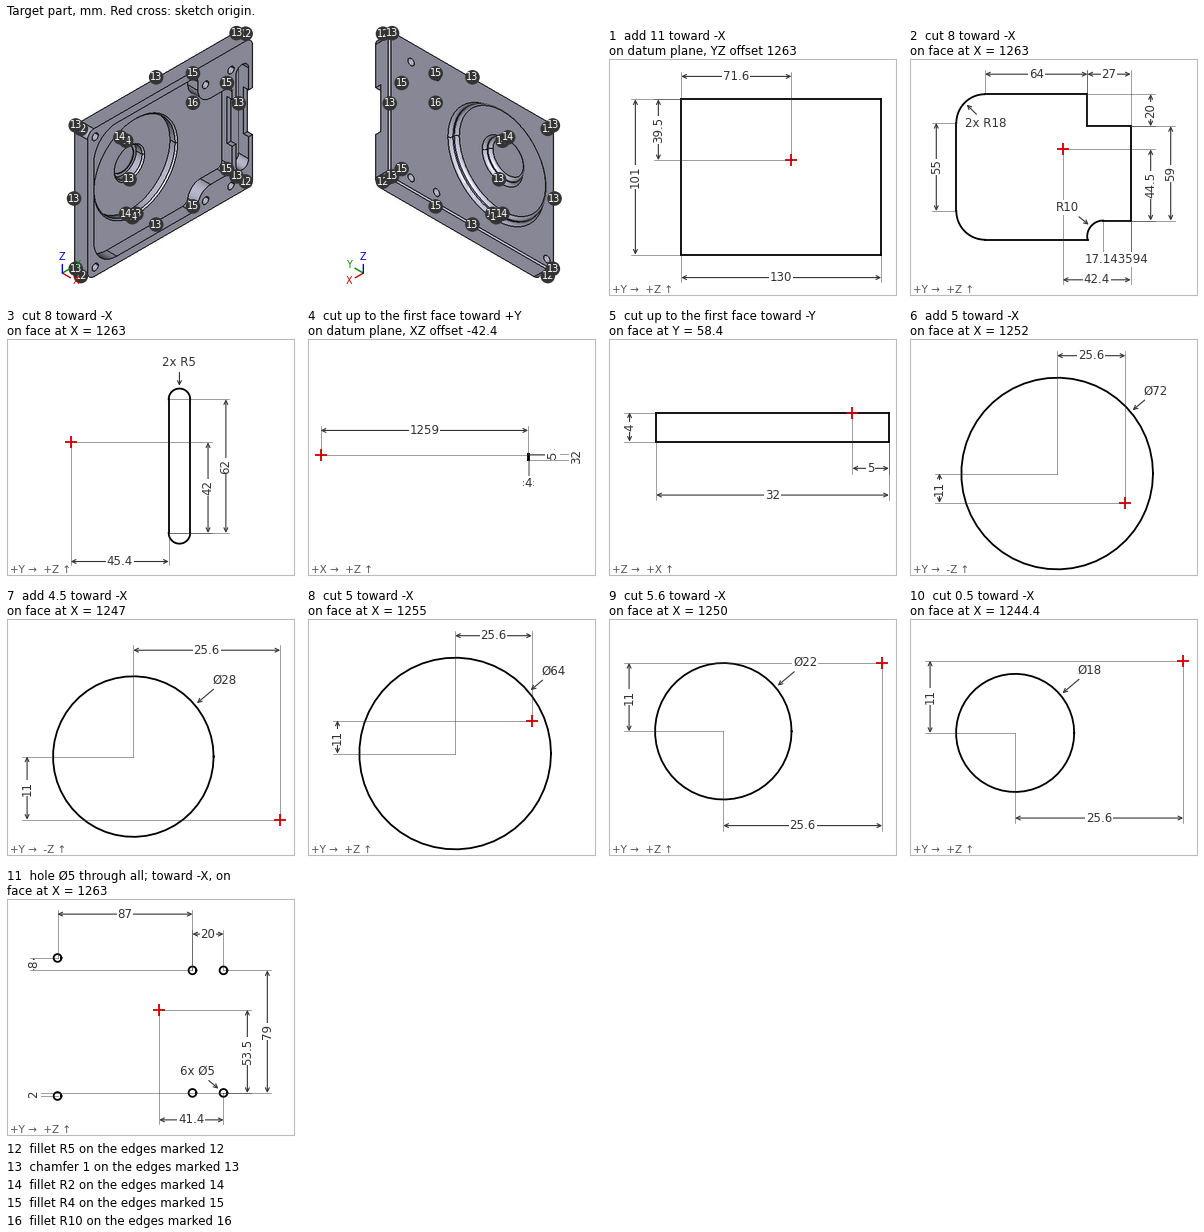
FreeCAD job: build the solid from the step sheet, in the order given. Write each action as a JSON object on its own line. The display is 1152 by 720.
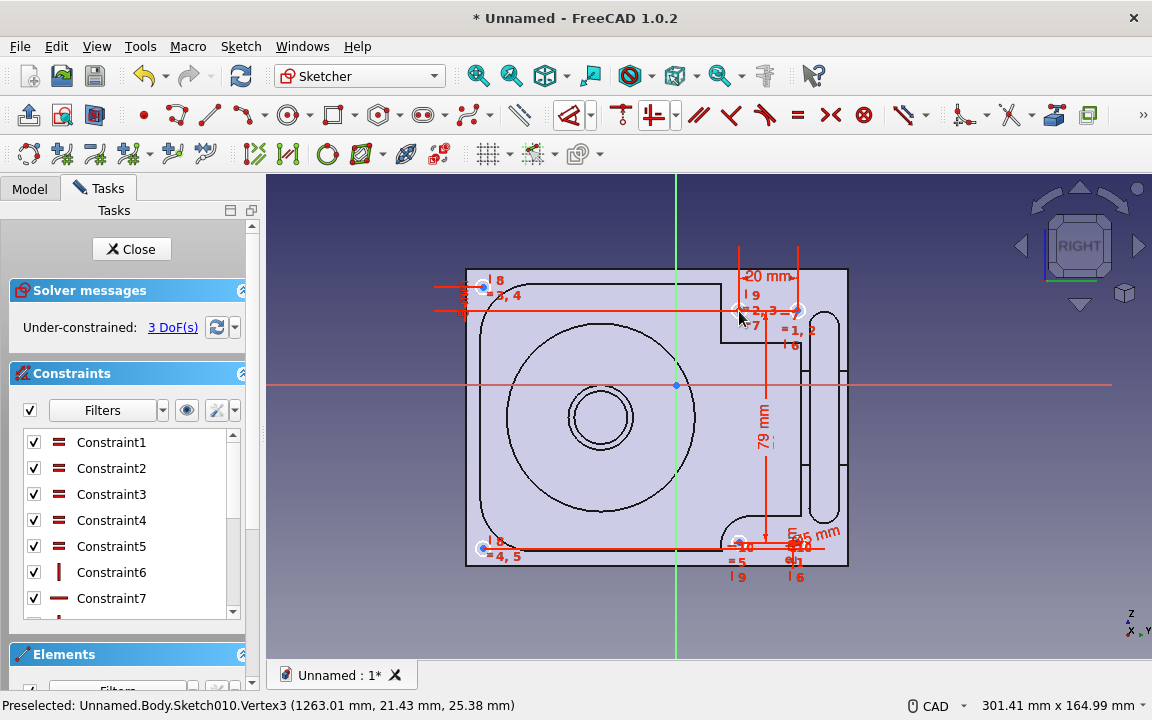
{"action": "left_click", "coordinate": [483, 287]}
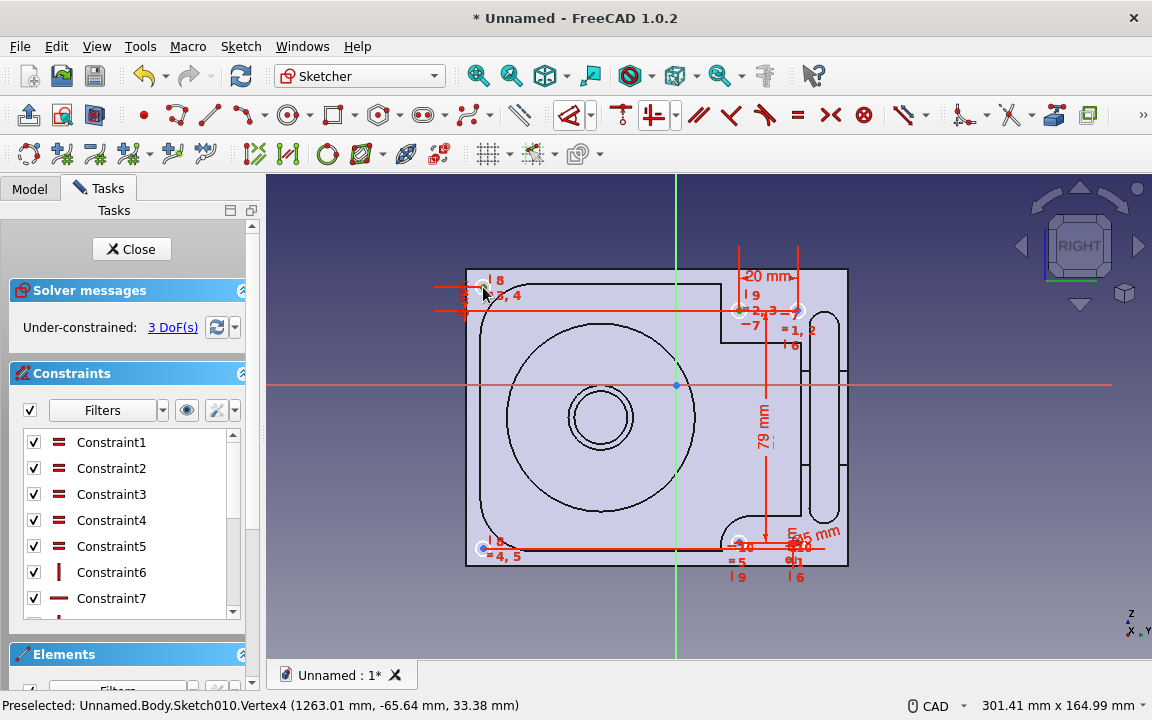
{"action": "key", "text": "l"}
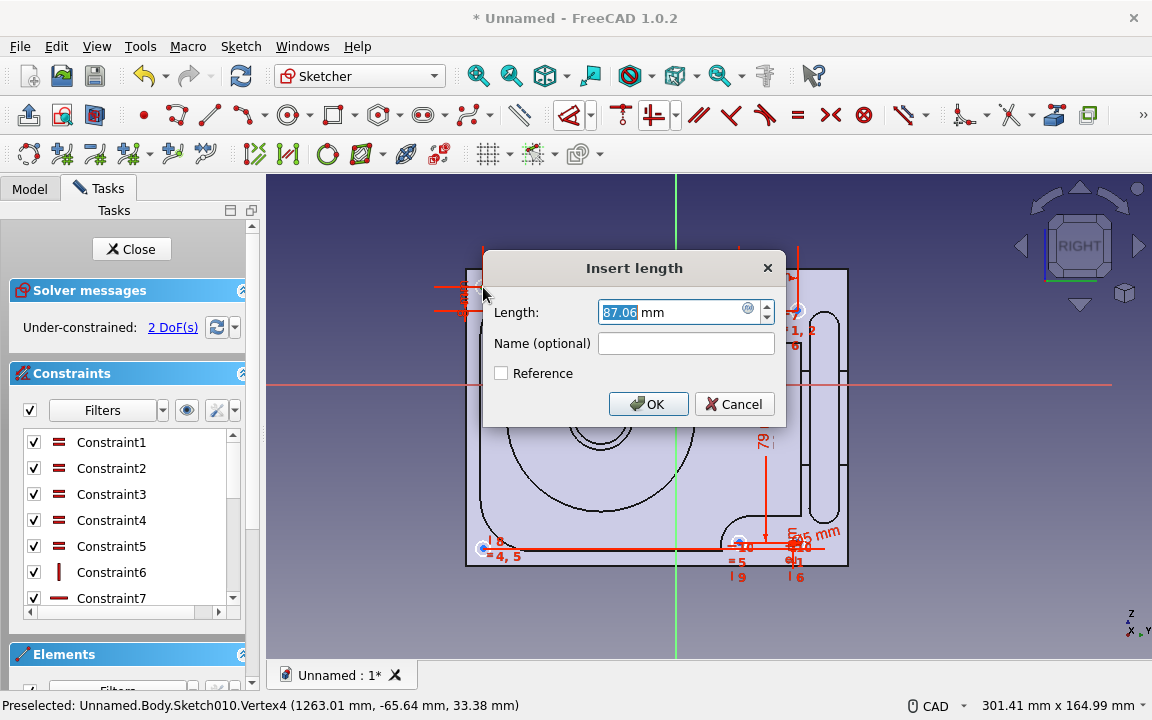
{"action": "type", "text": "87"}
{"action": "key", "text": "Return"}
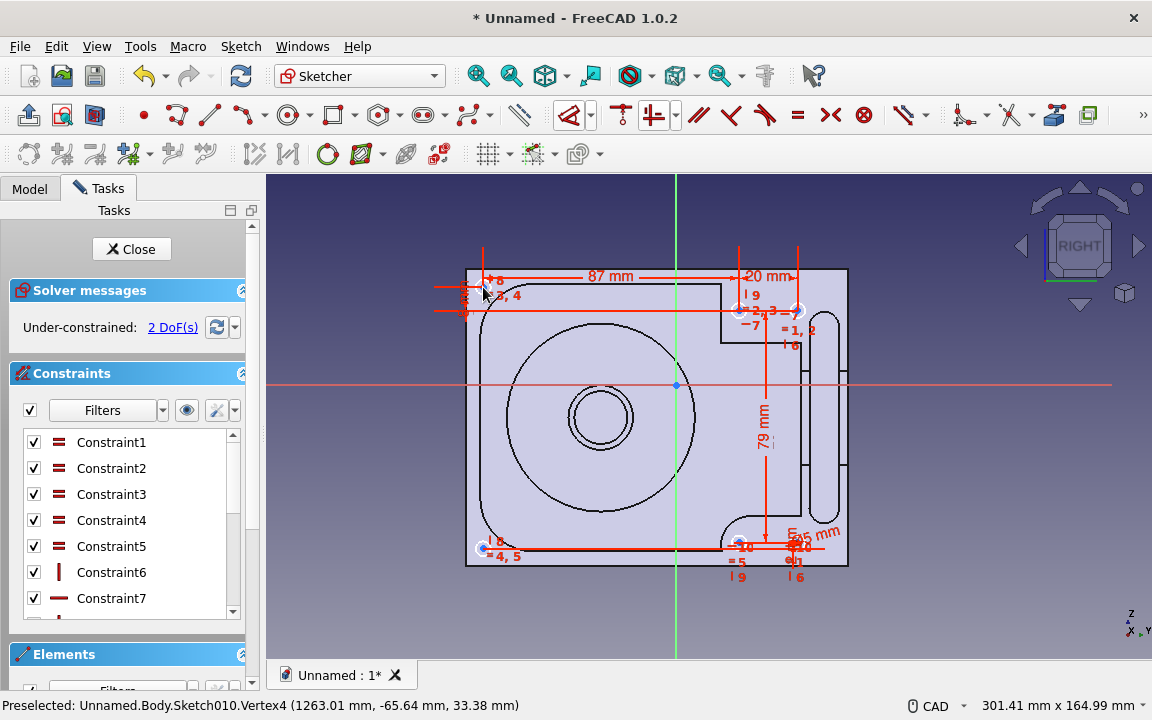
{"action": "left_click", "coordinate": [798, 543]}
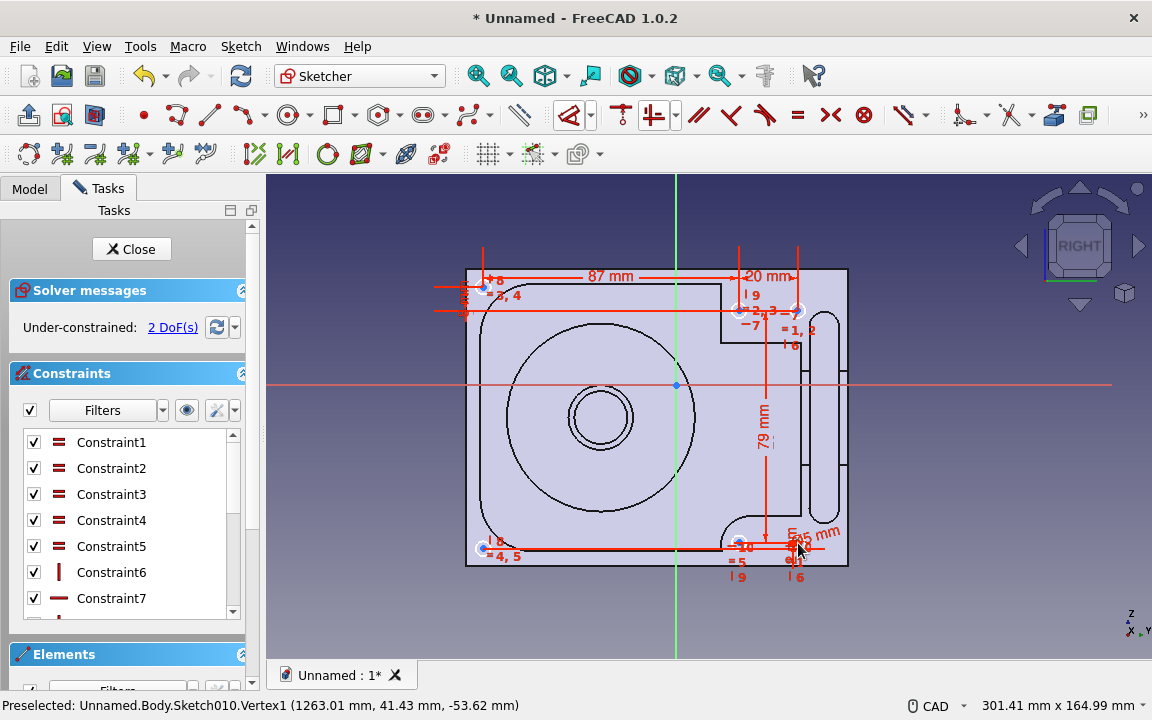
{"action": "key", "text": "l"}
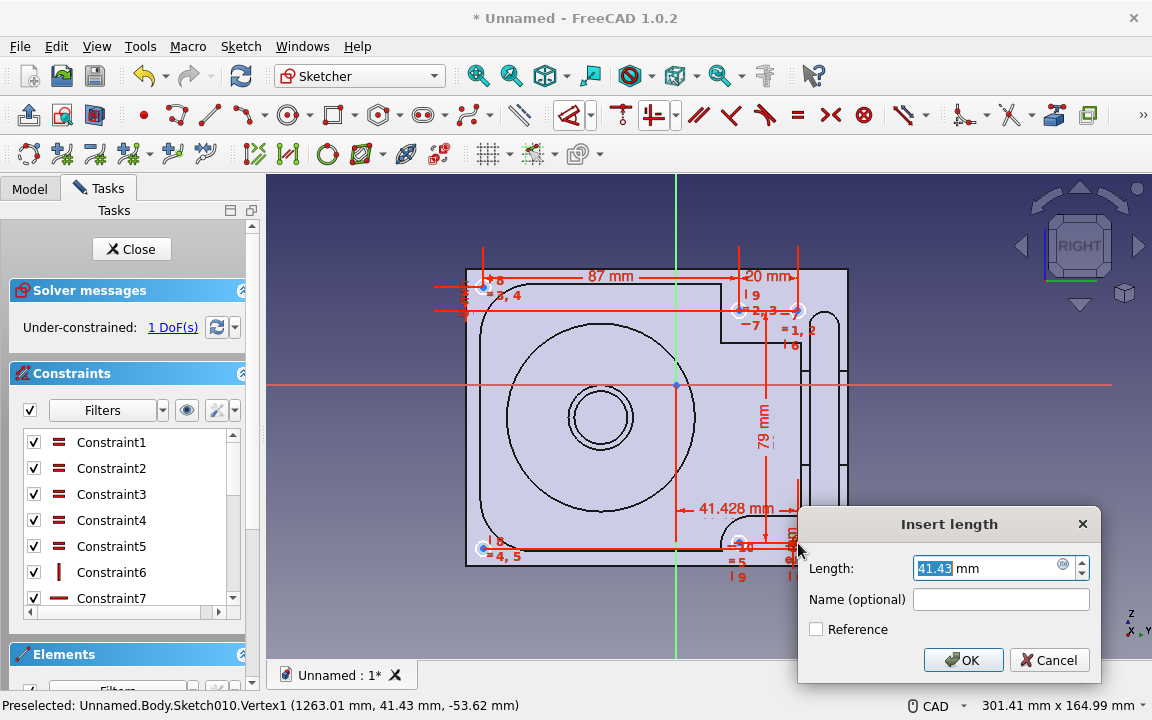
{"action": "type", "text": "41.4"}
{"action": "key", "text": "Return"}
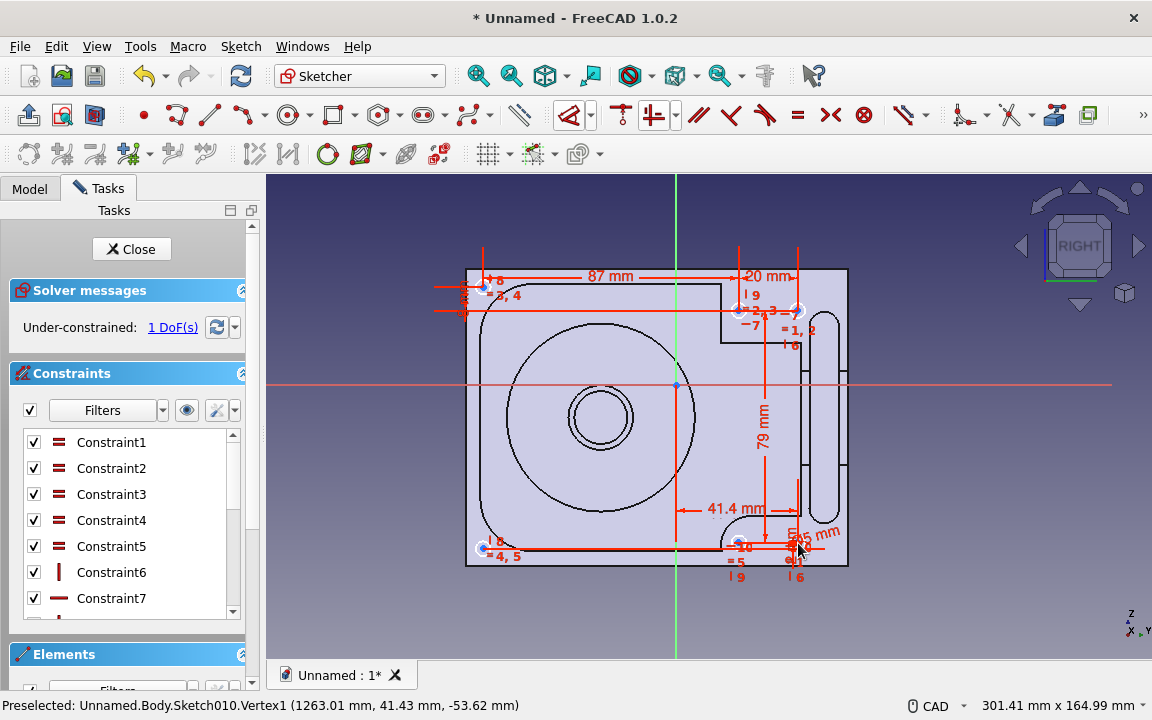
{"action": "left_click", "coordinate": [798, 543]}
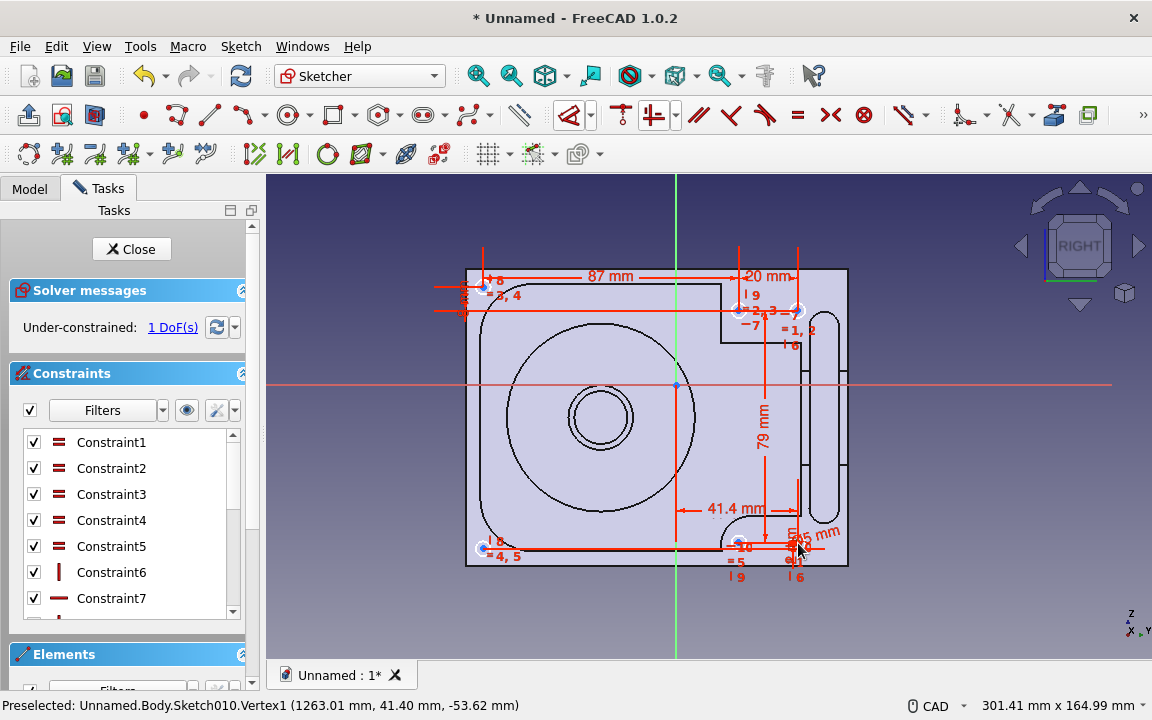
{"action": "key", "text": "i"}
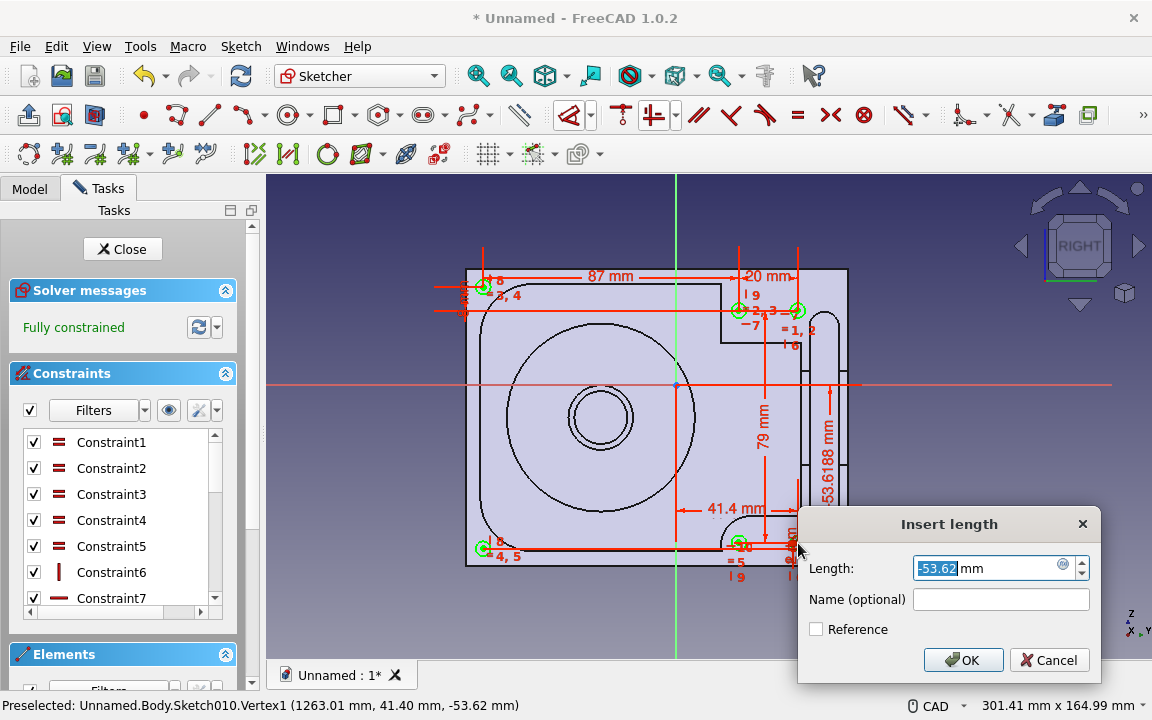
{"action": "type", "text": "-53.5"}
{"action": "key", "text": "Return"}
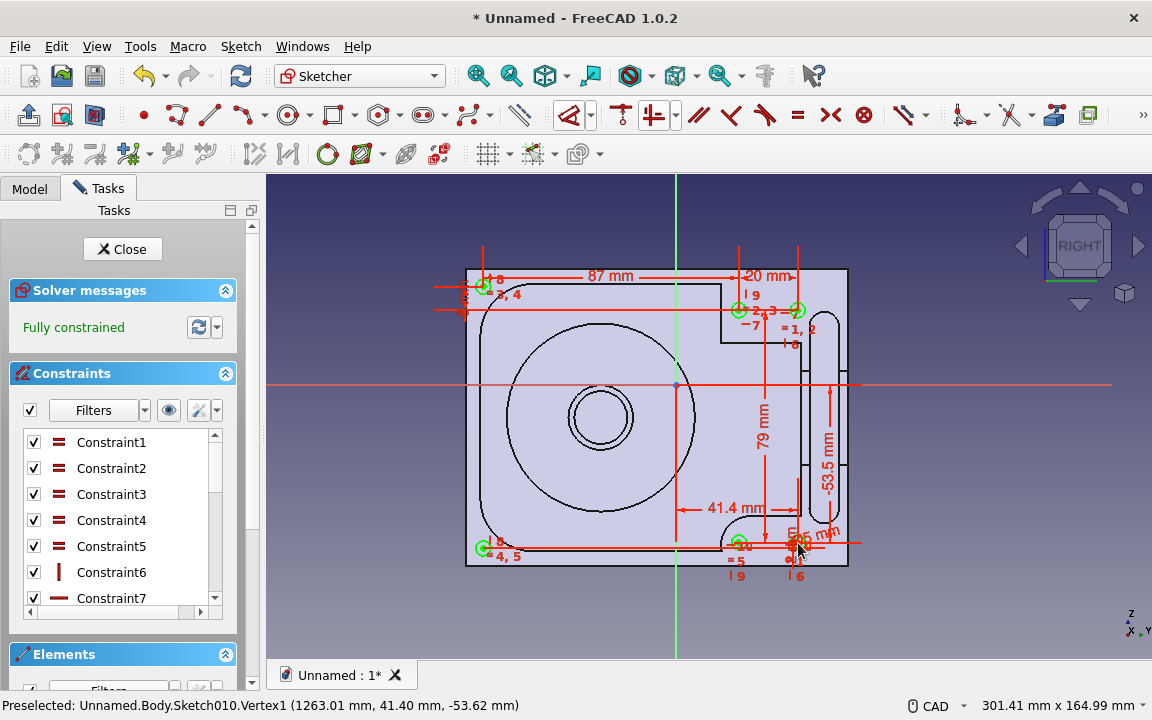
{"action": "left_click", "coordinate": [123, 249]}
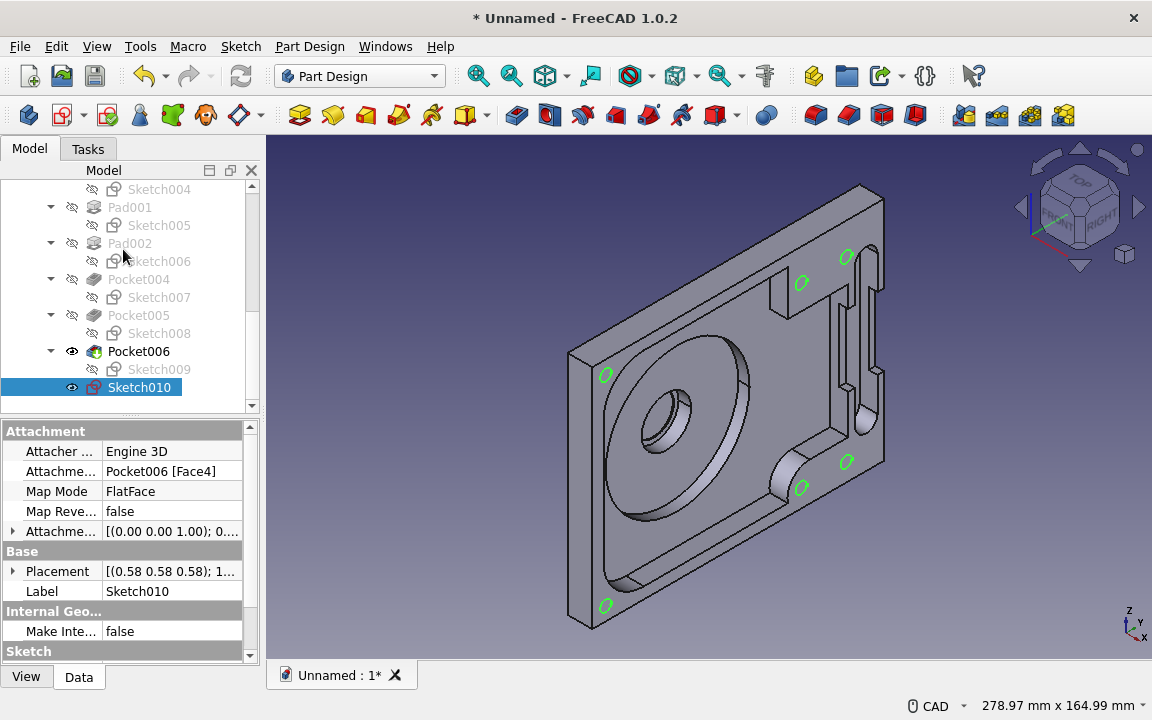
{"action": "left_click", "coordinate": [550, 116]}